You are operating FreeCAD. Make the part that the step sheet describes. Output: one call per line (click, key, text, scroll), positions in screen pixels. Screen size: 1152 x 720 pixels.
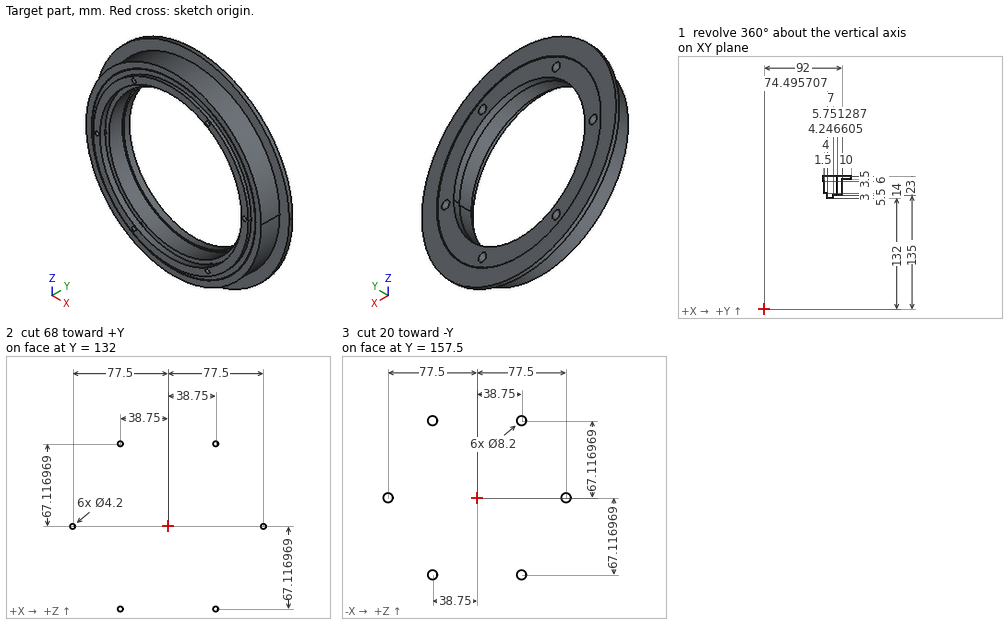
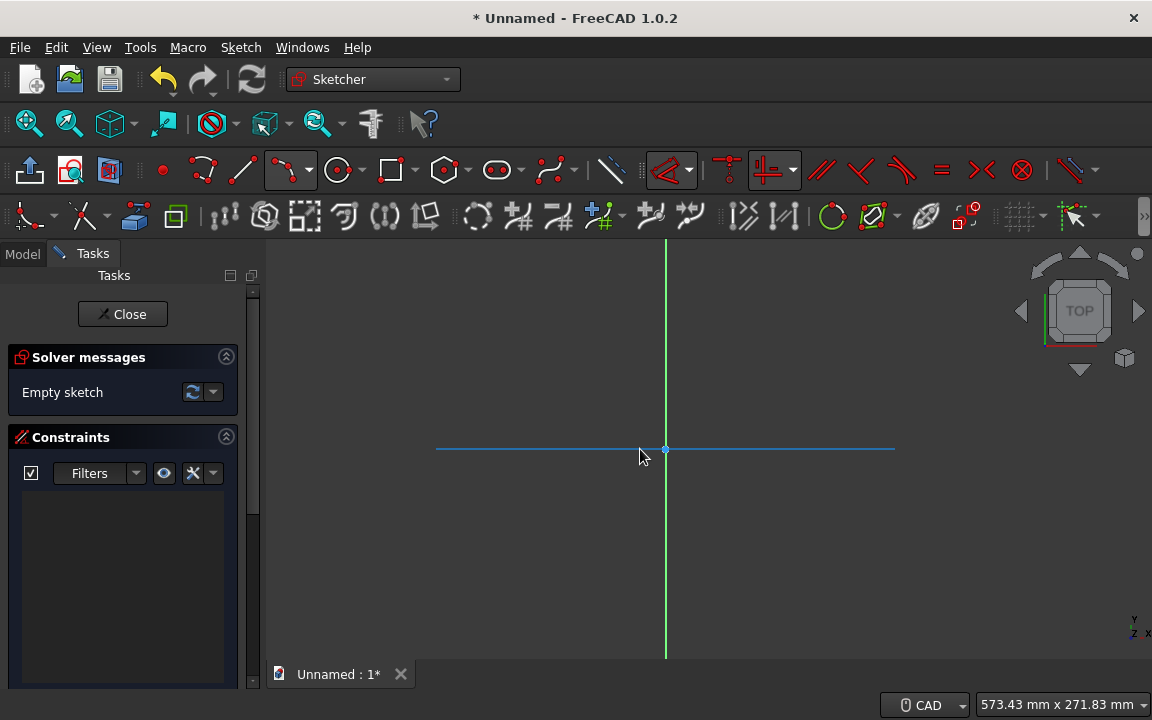
scroll(640, 449, down, 5)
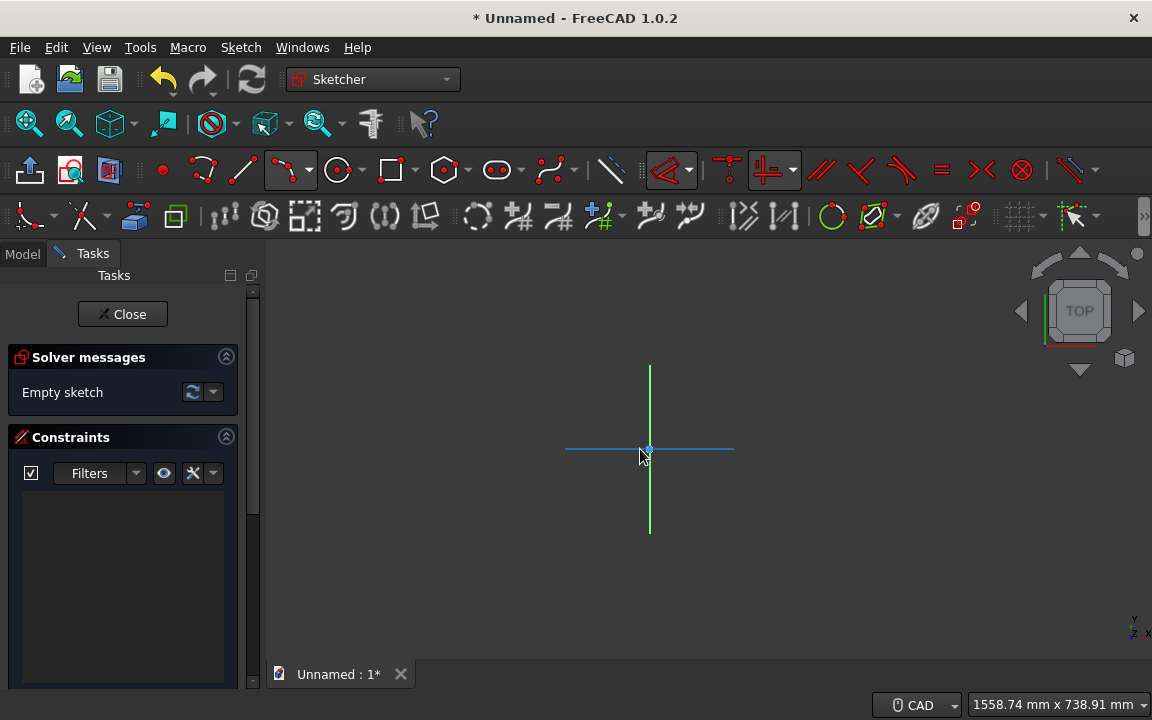
scroll(702, 362, up, 14)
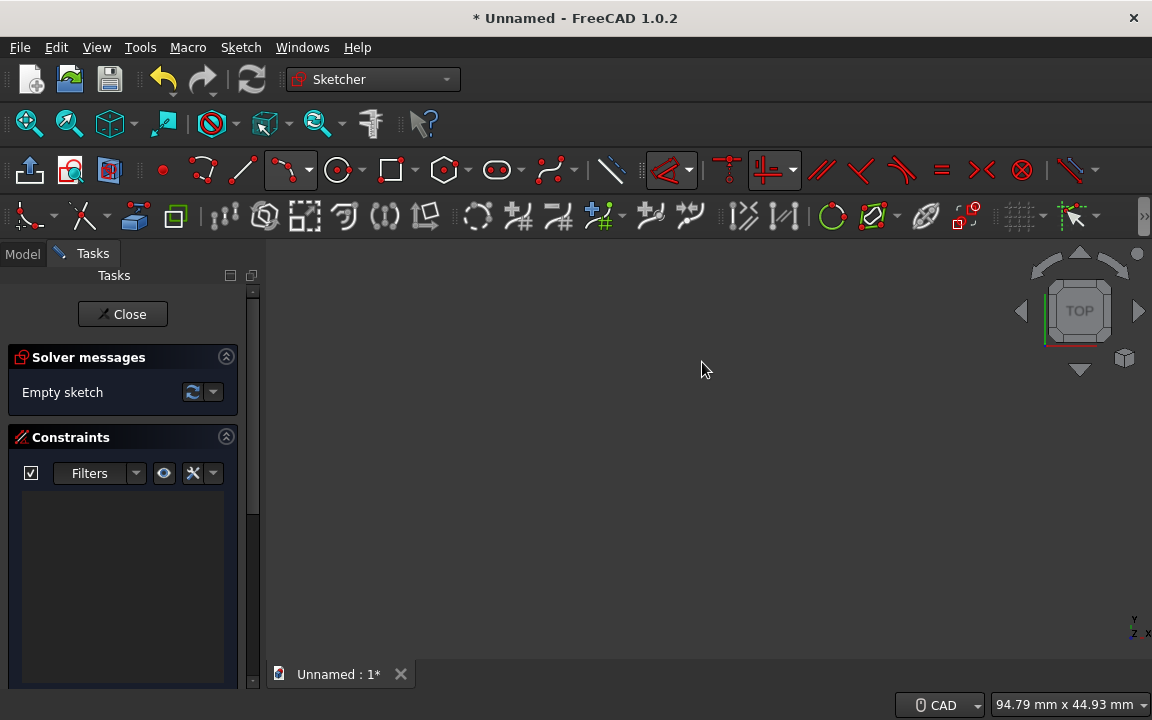
click(204, 170)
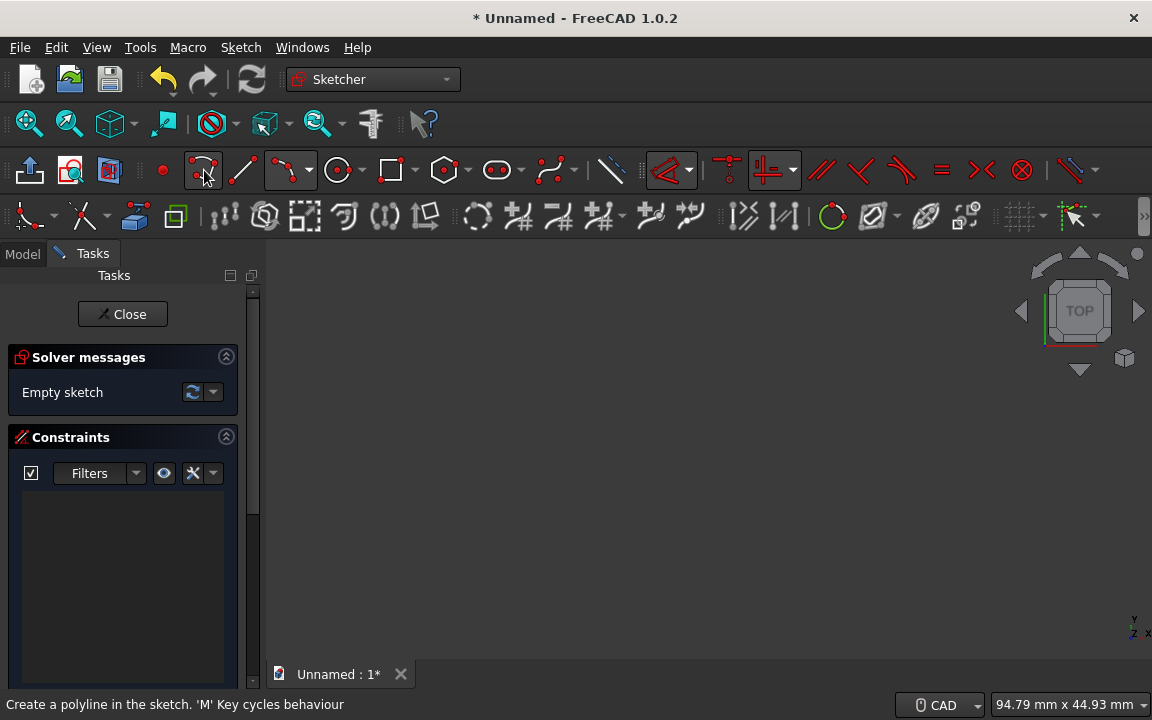
click(641, 533)
click(694, 533)
click(694, 351)
click(788, 351)
click(788, 318)
click(641, 318)
click(641, 534)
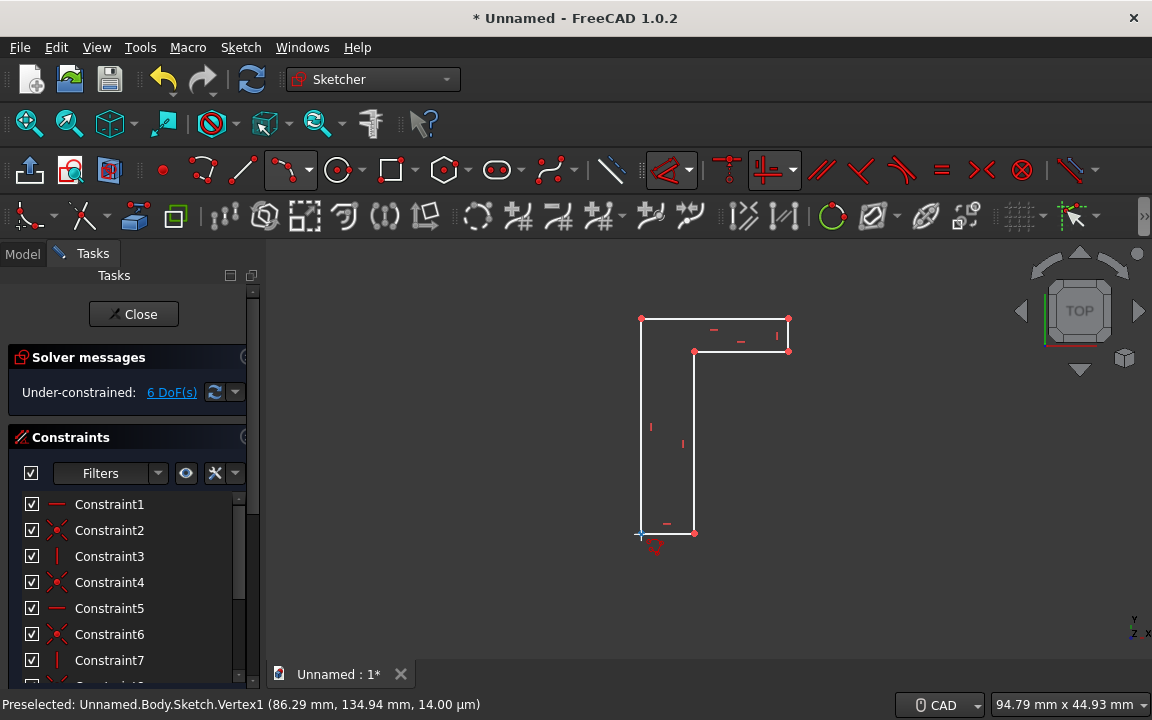
click(531, 561)
click(596, 561)
click(596, 533)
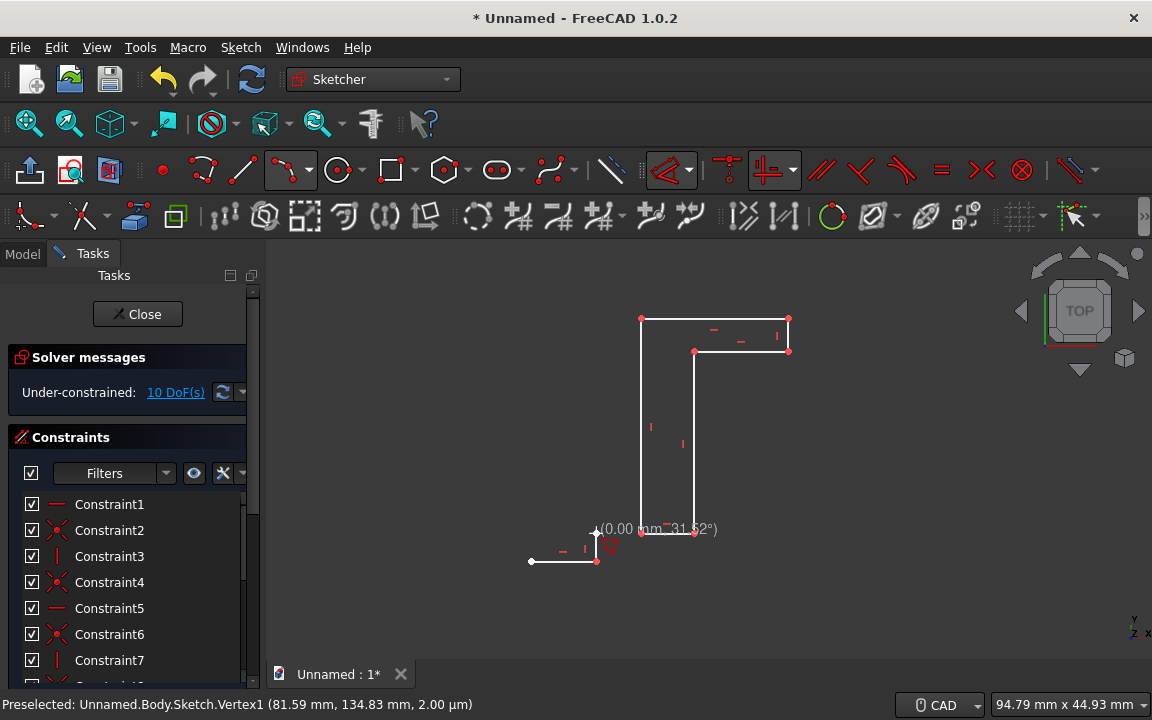
scroll(636, 533, up, 7)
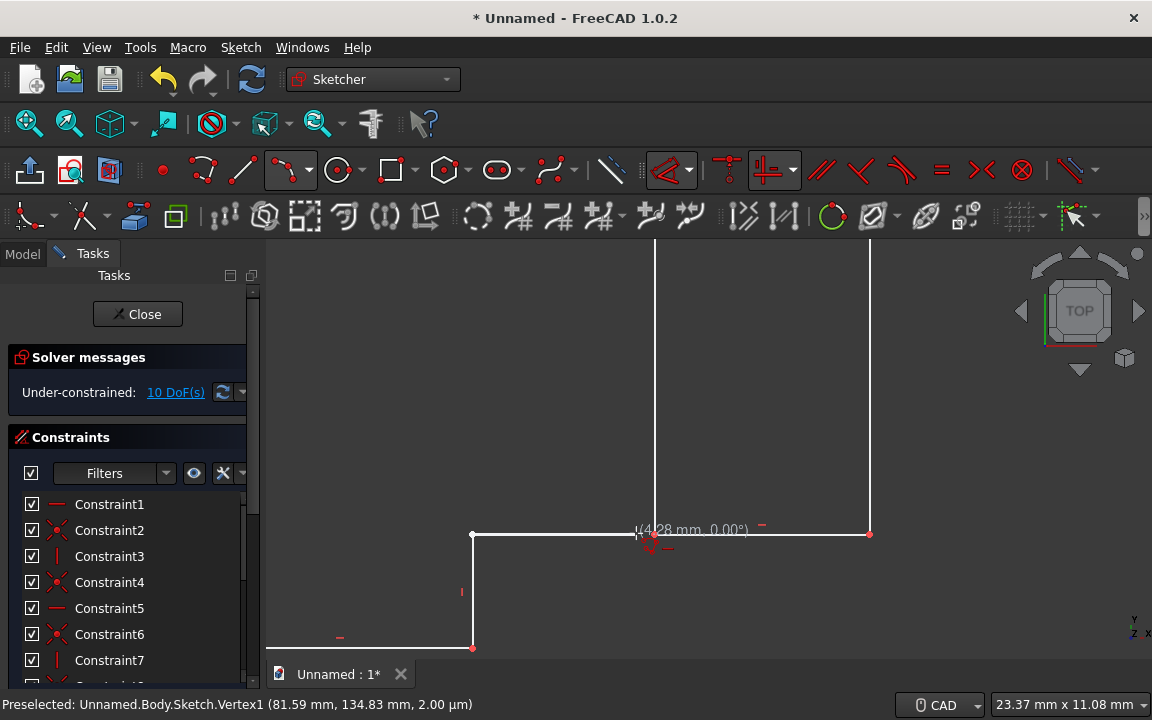
click(634, 531)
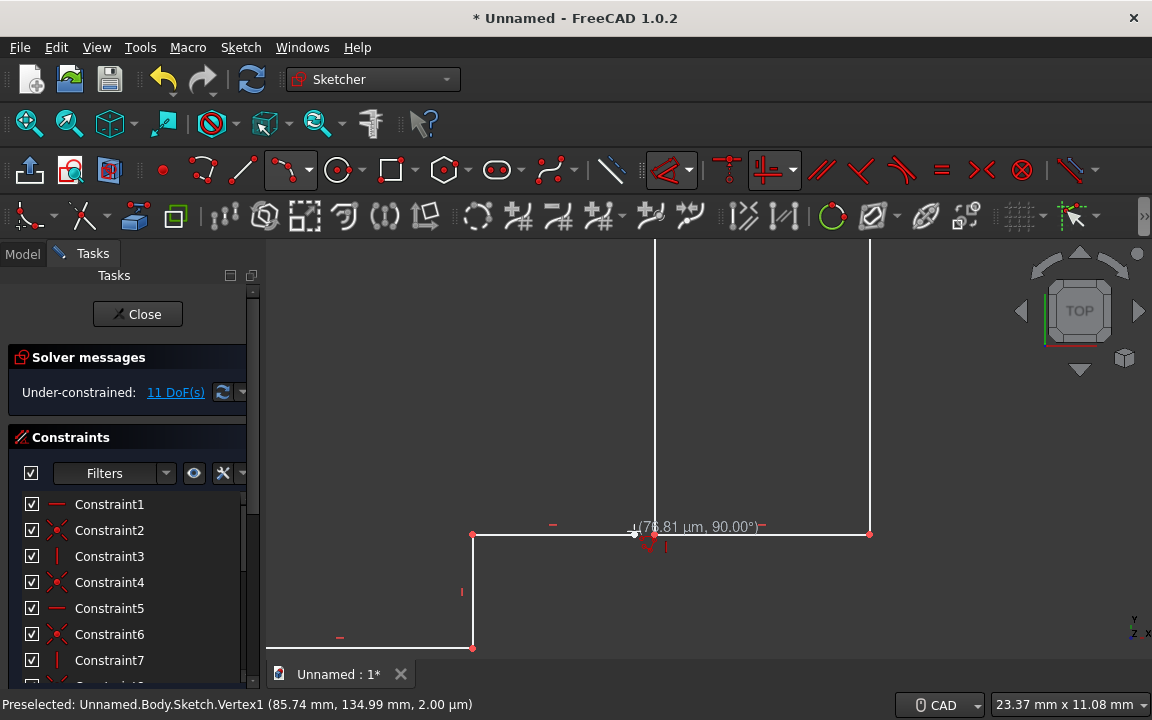
scroll(646, 546, down, 7)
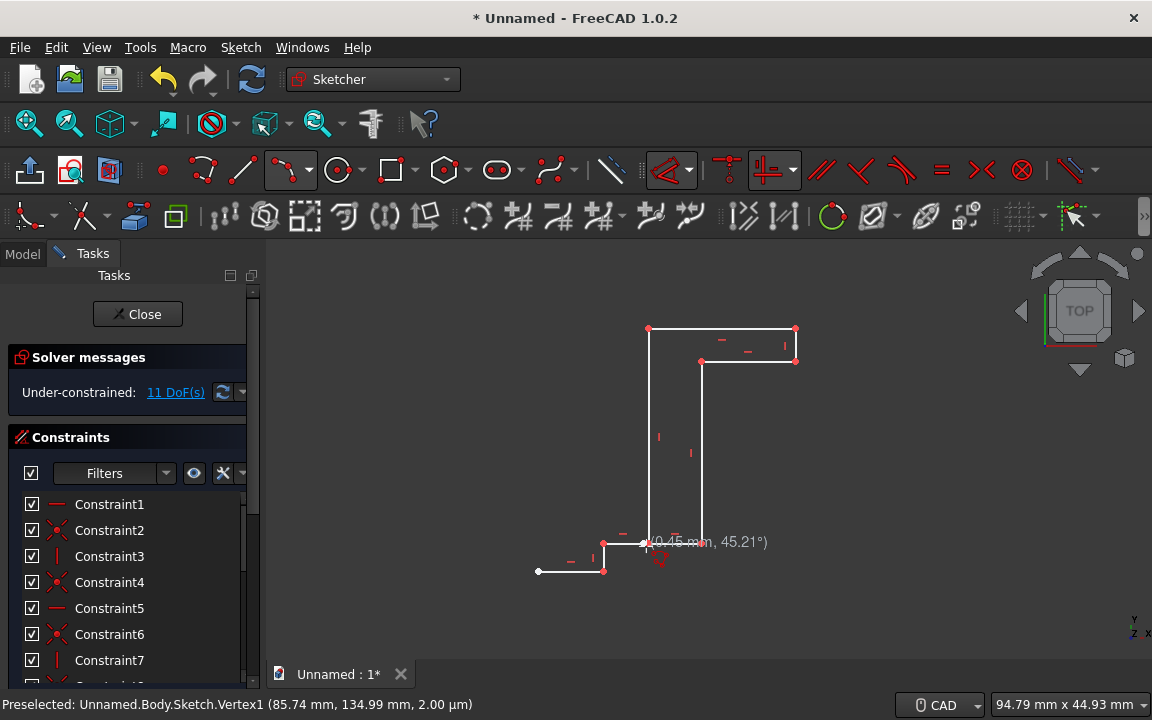
scroll(643, 333, up, 7)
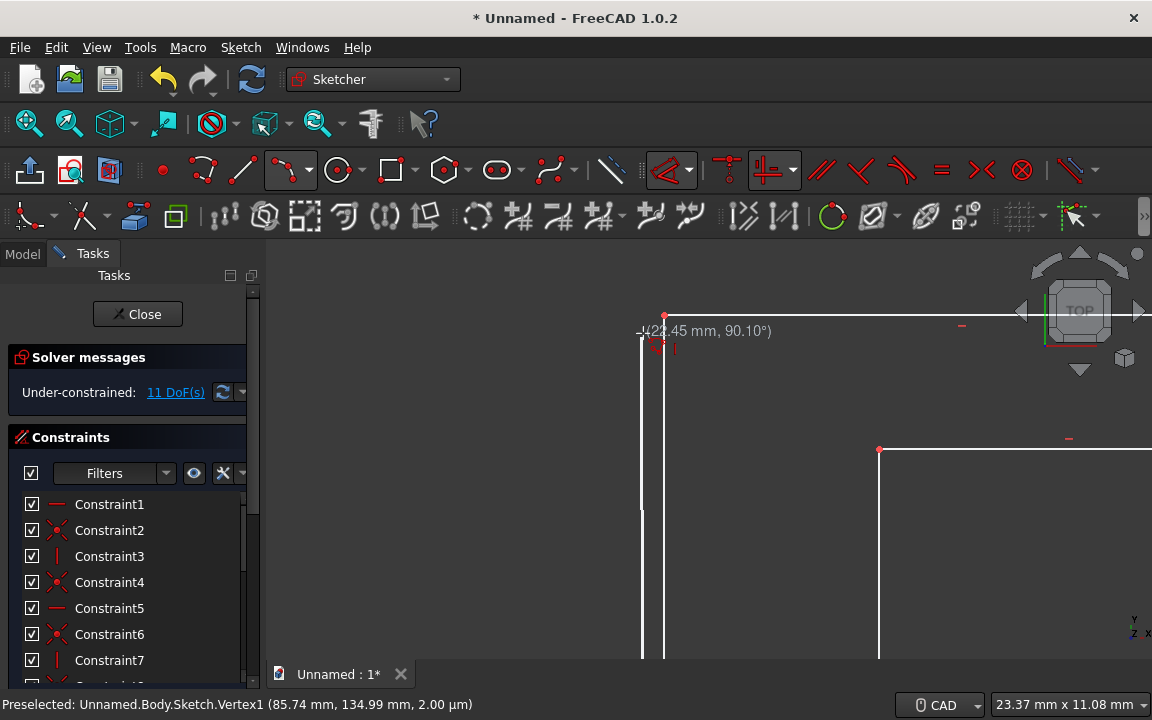
click(643, 332)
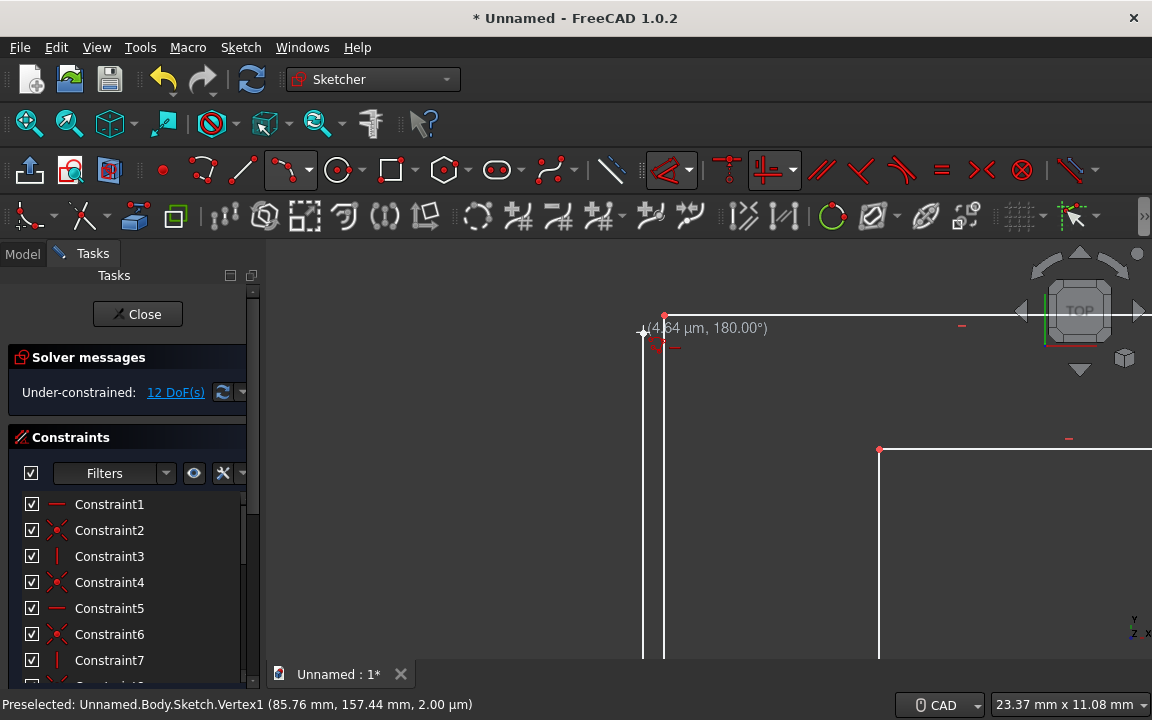
scroll(643, 332, down, 7)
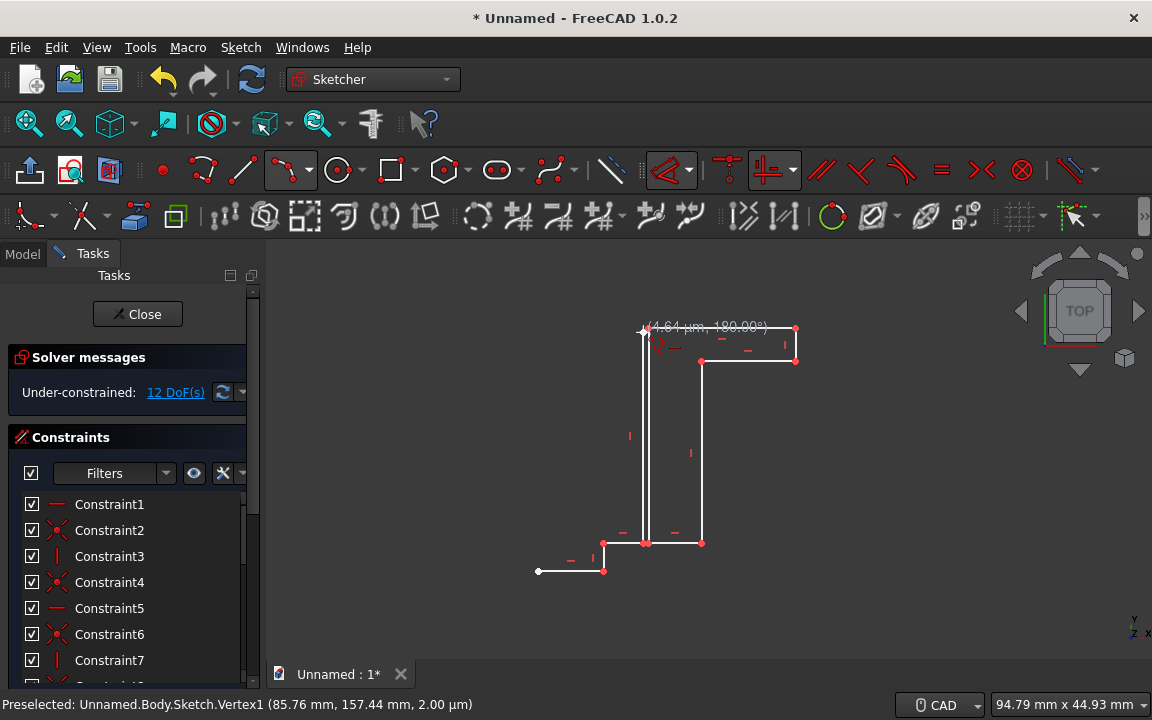
click(487, 332)
click(487, 388)
click(501, 388)
click(501, 519)
click(538, 519)
click(539, 571)
key(Escape)
key(Escape)